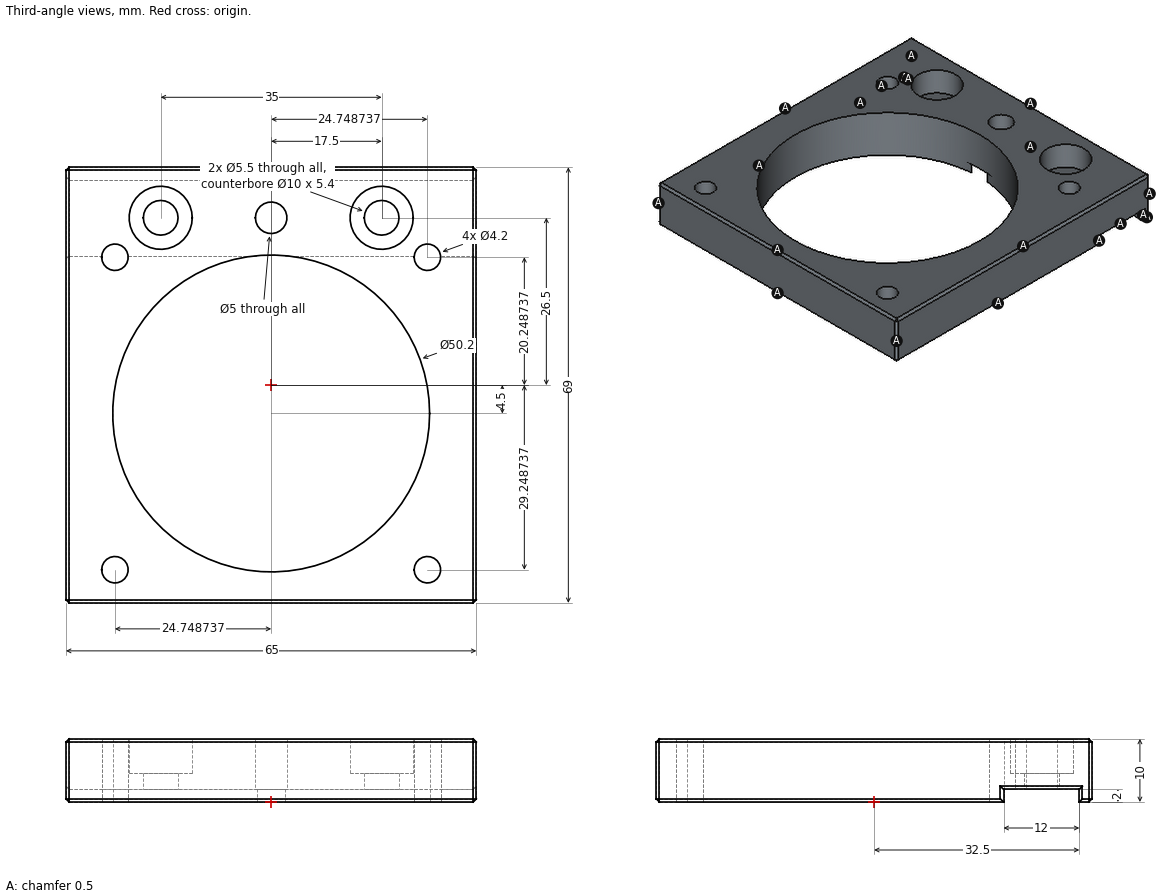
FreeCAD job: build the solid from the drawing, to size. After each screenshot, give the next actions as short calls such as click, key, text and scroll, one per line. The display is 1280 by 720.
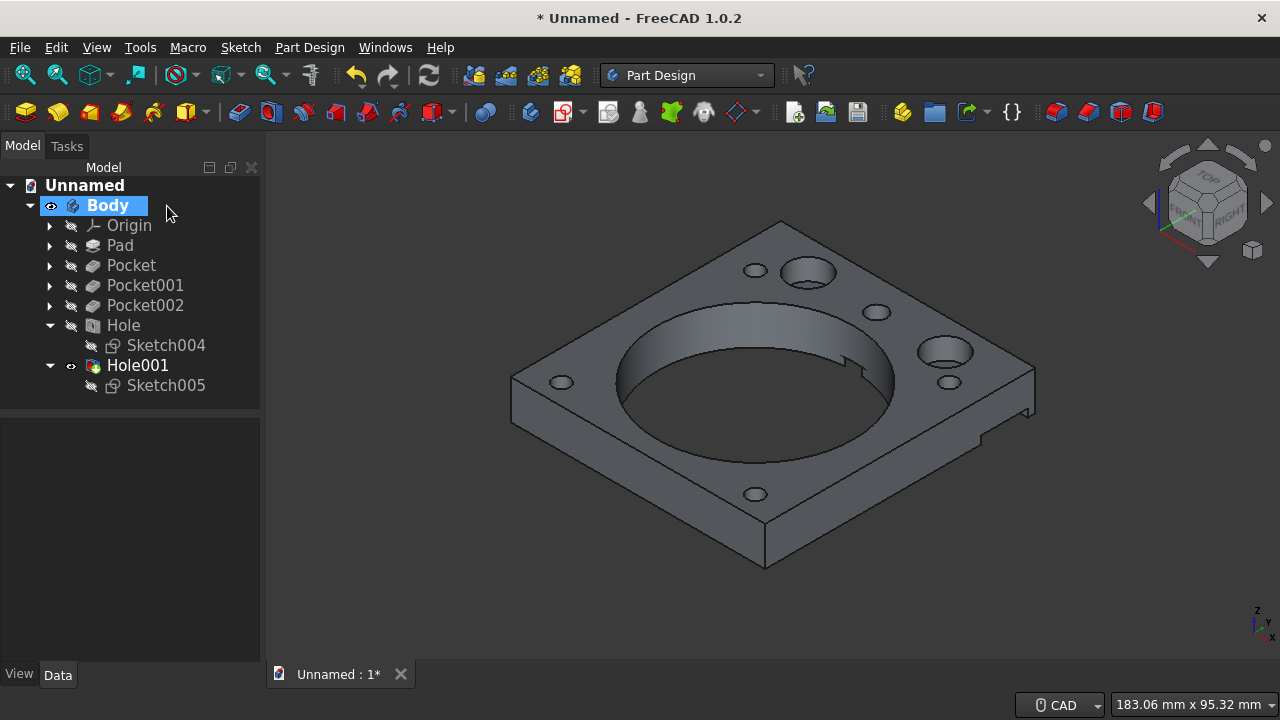
click(939, 445)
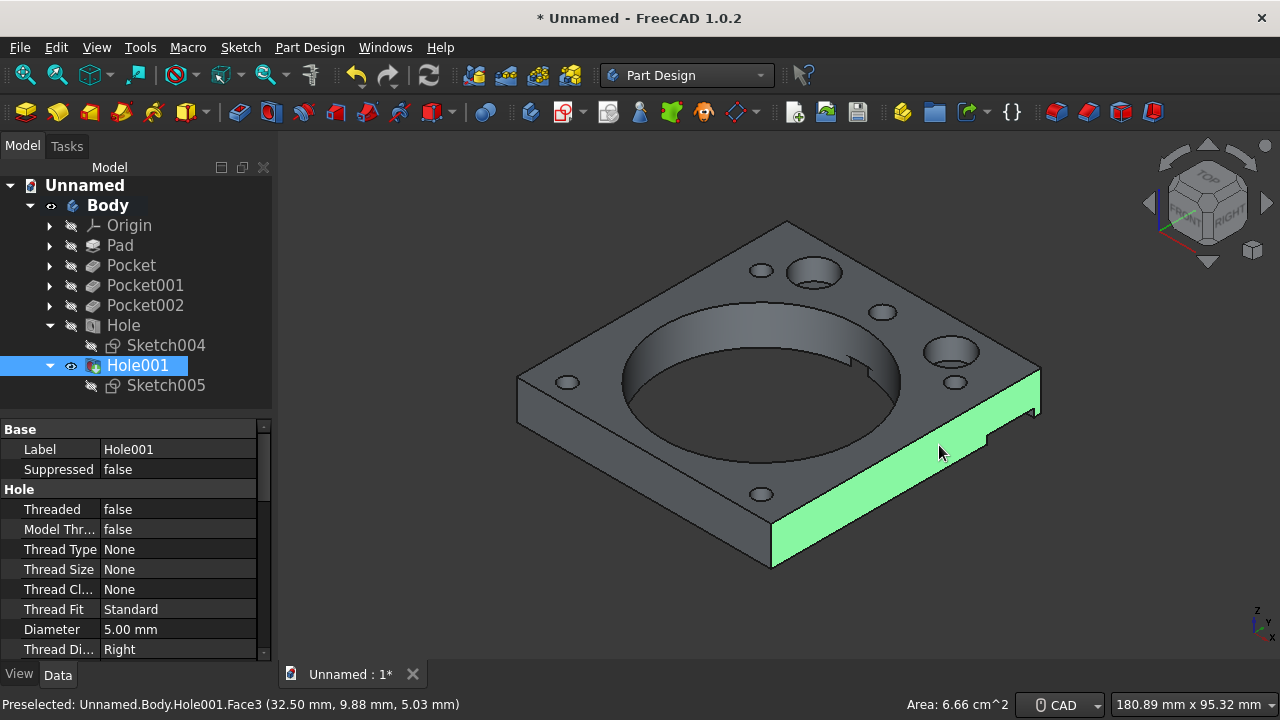
click(644, 449, ctrl)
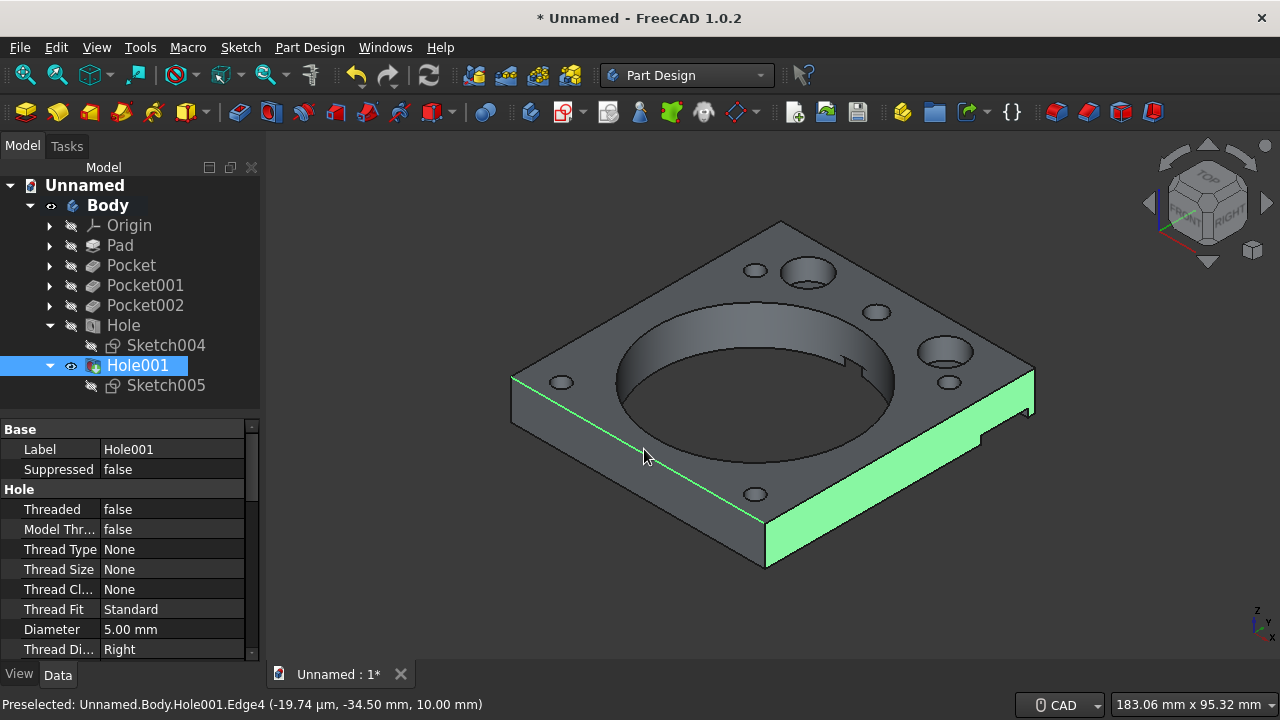
key(2)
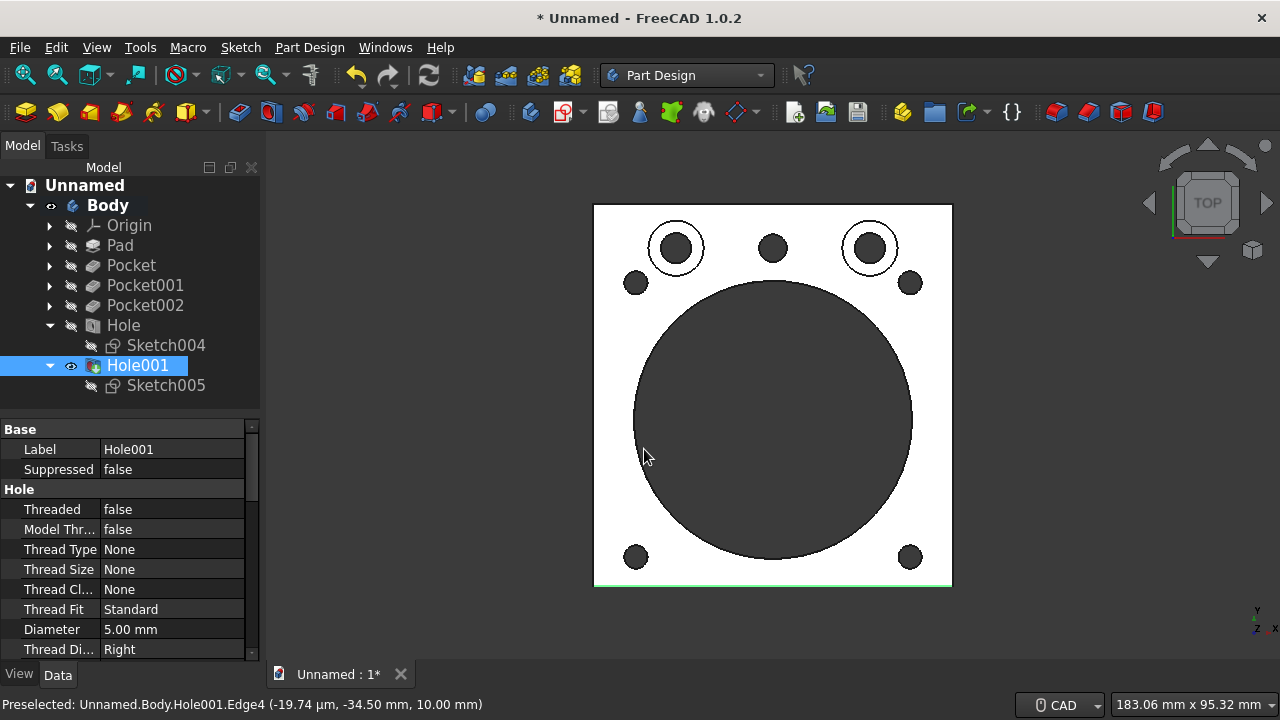
click(773, 203, ctrl)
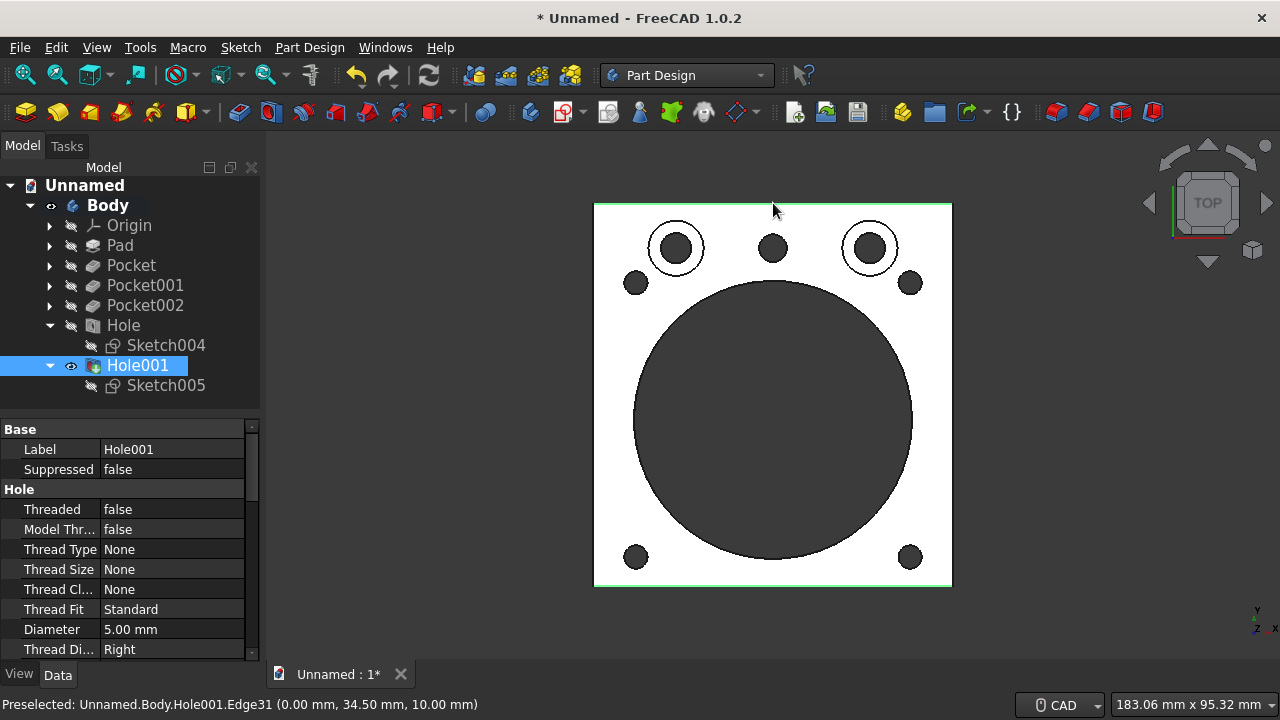
key(0)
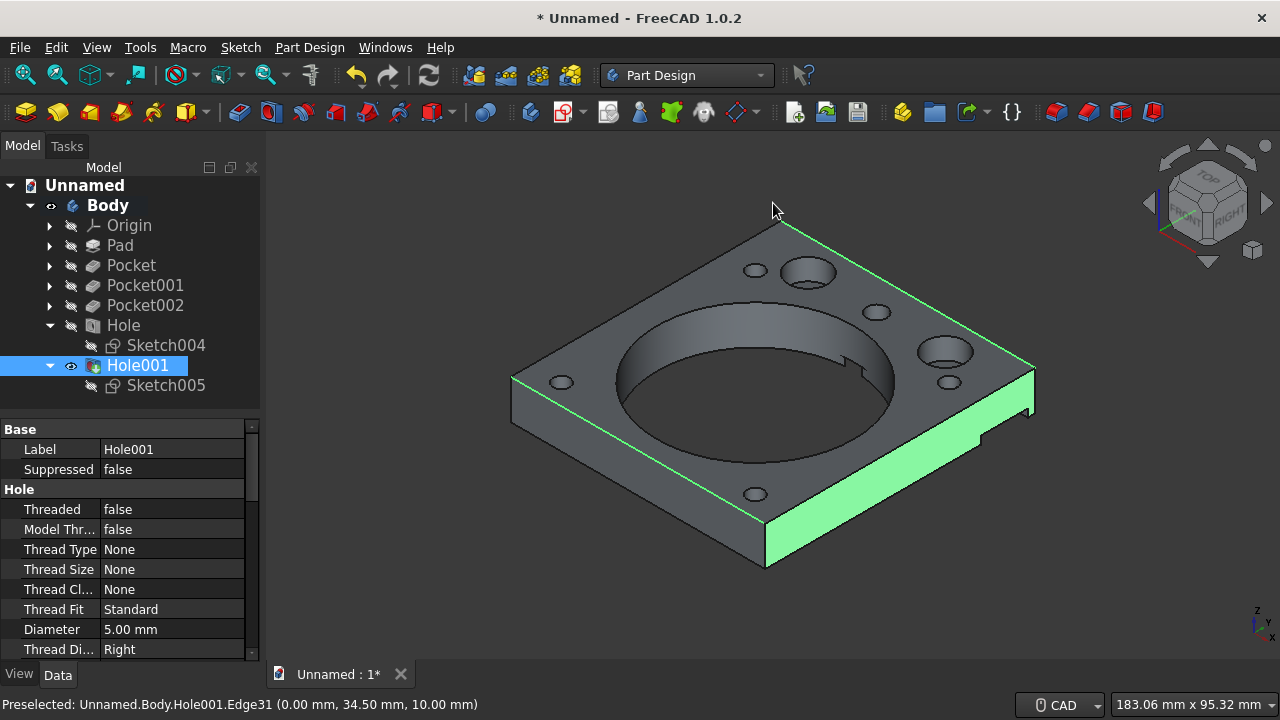
key(1)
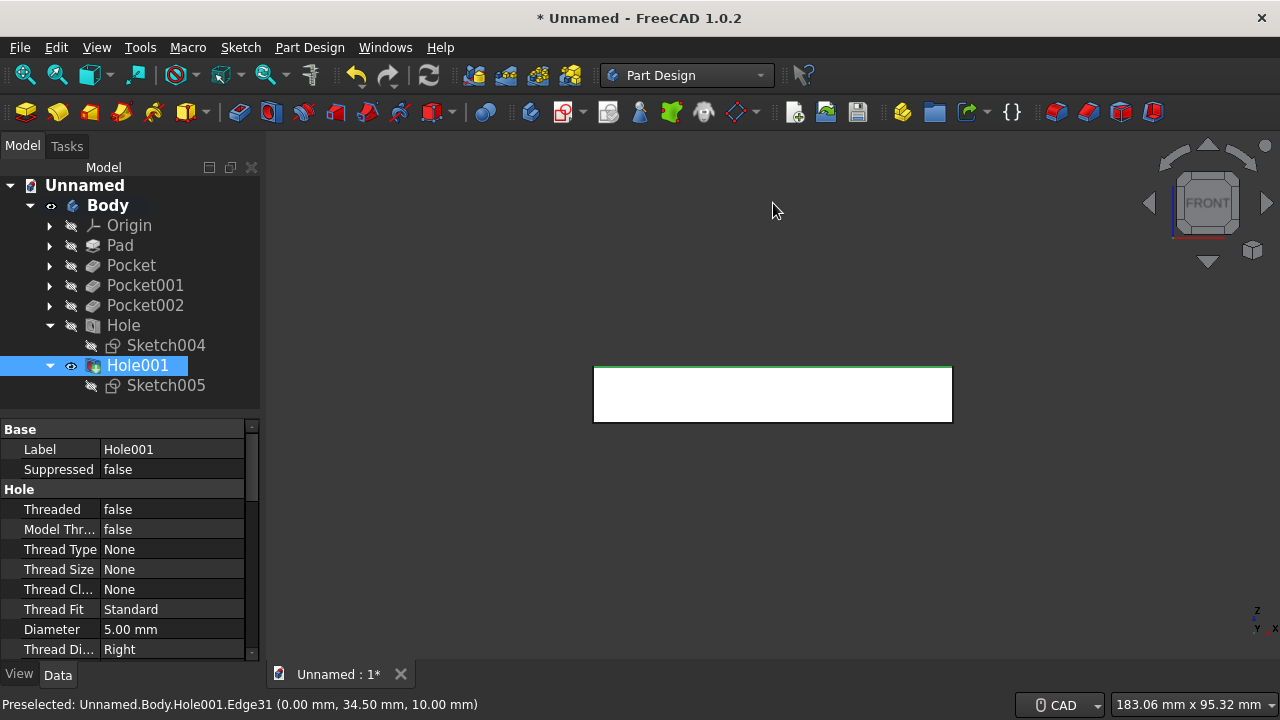
click(26, 76)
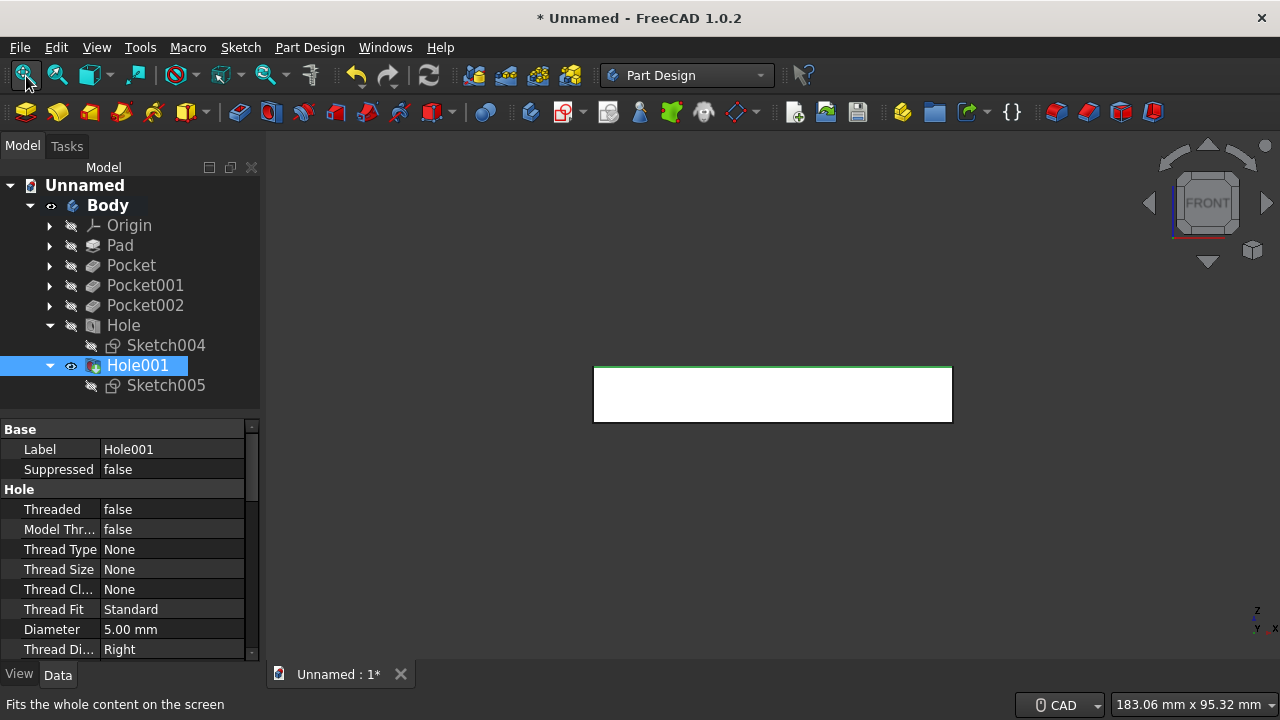
click(773, 422, ctrl)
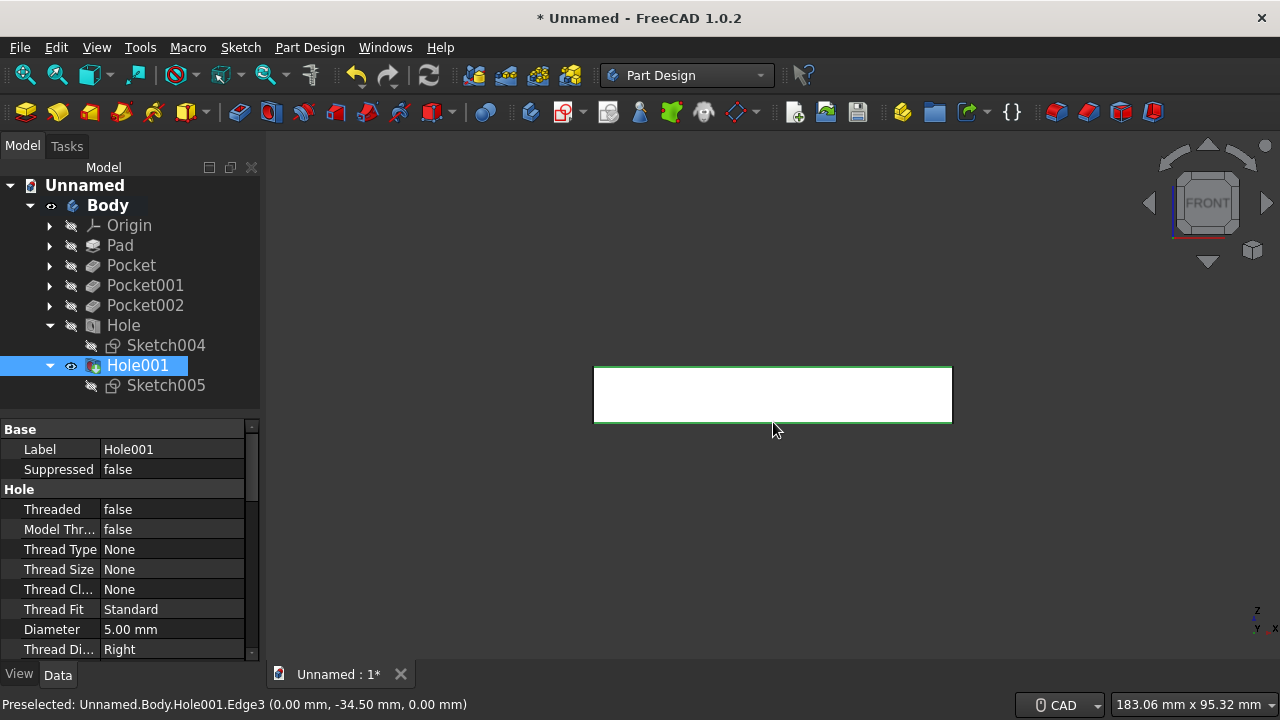
key(3)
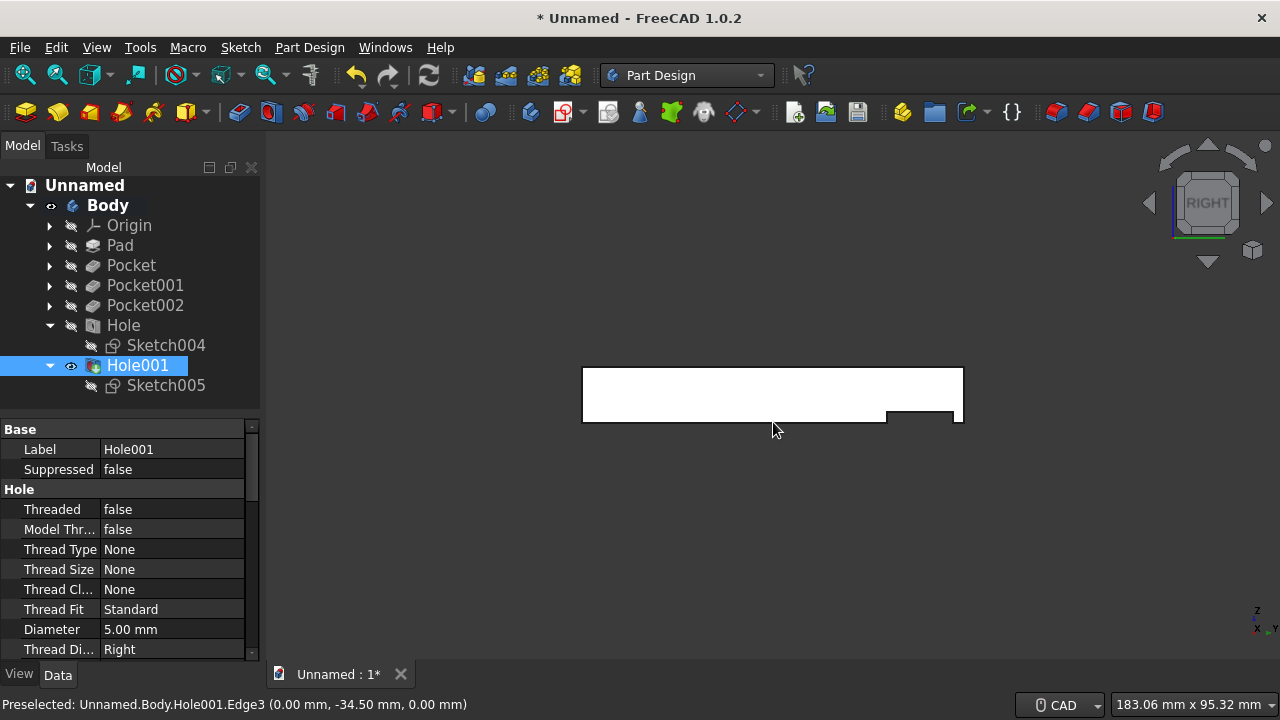
click(26, 76)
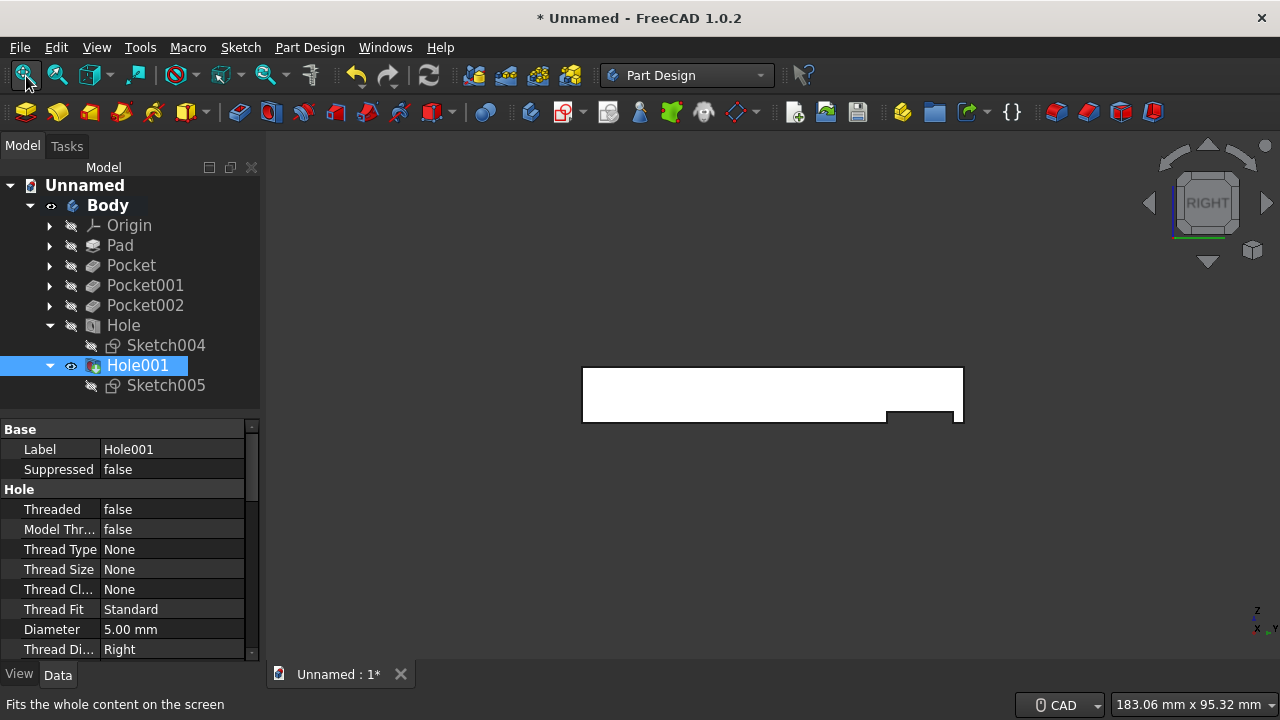
key(5)